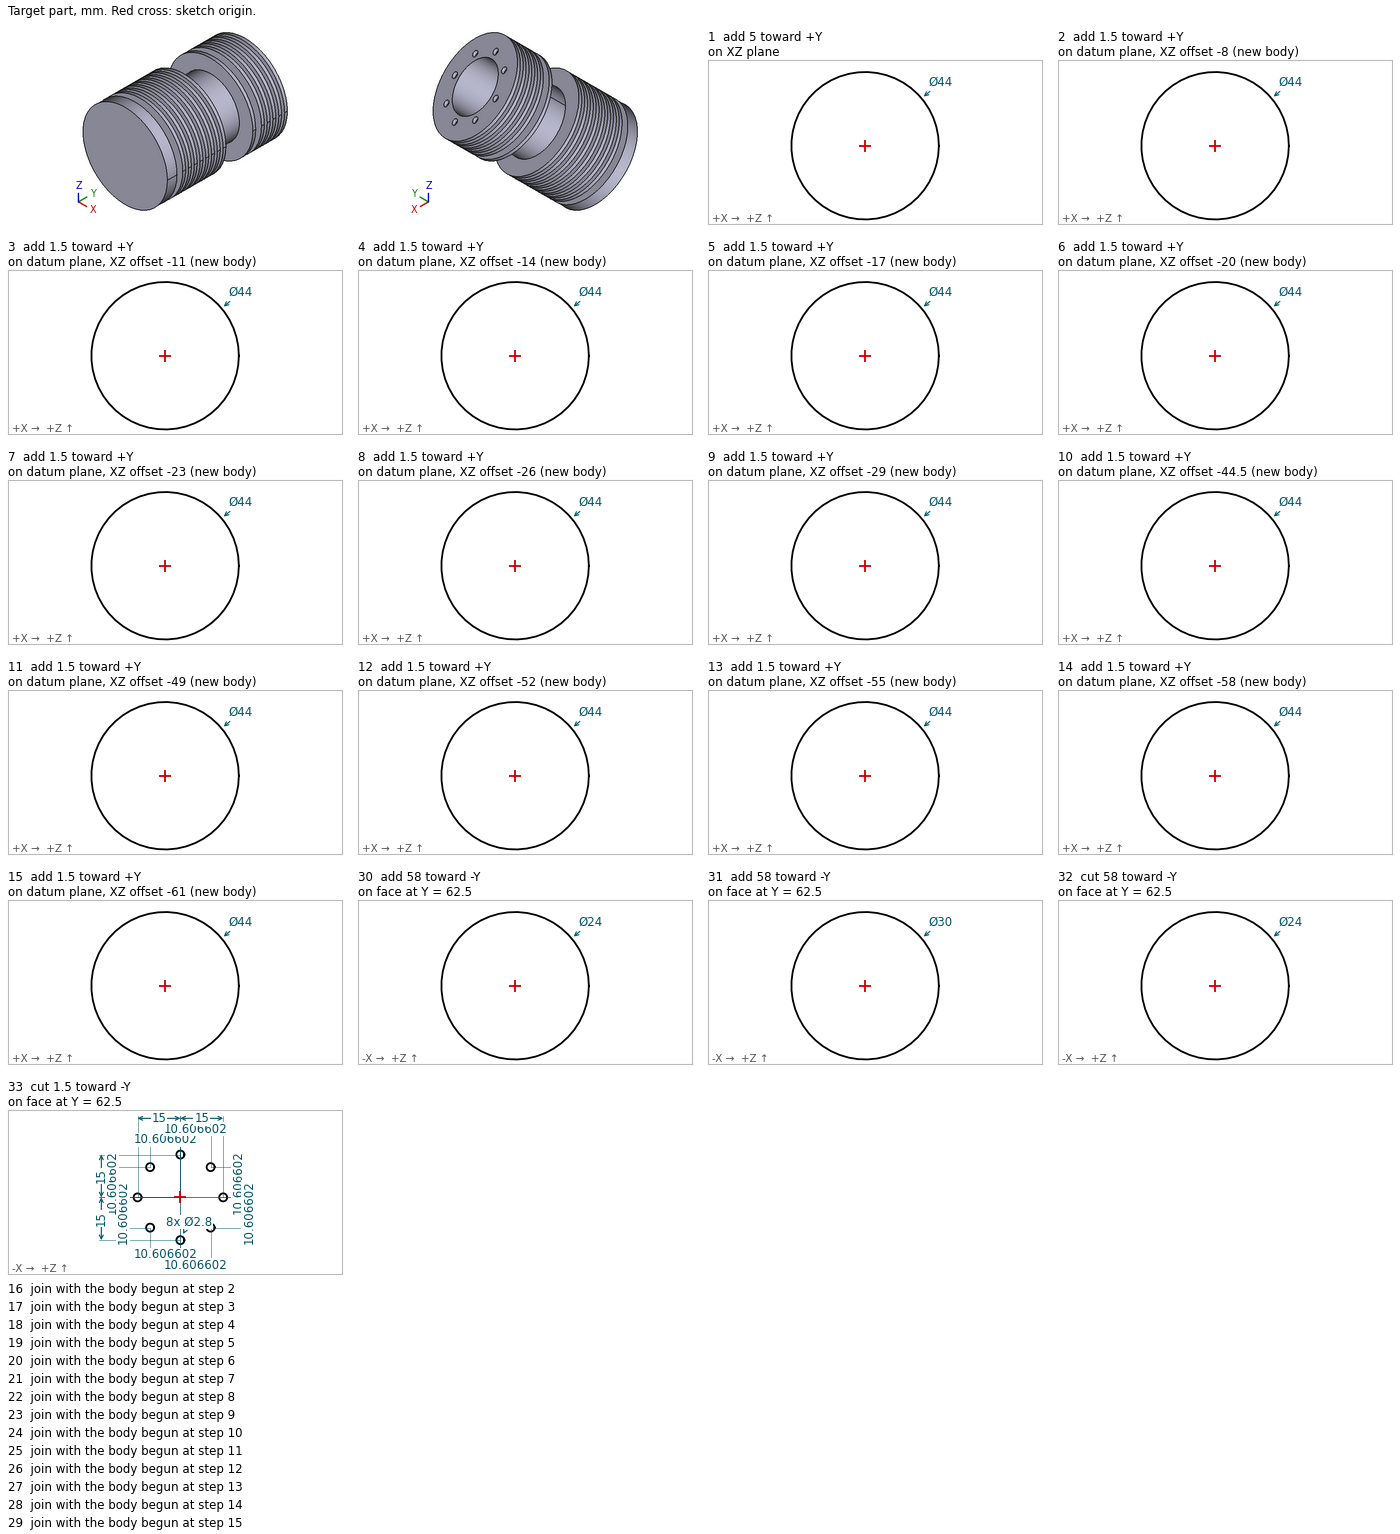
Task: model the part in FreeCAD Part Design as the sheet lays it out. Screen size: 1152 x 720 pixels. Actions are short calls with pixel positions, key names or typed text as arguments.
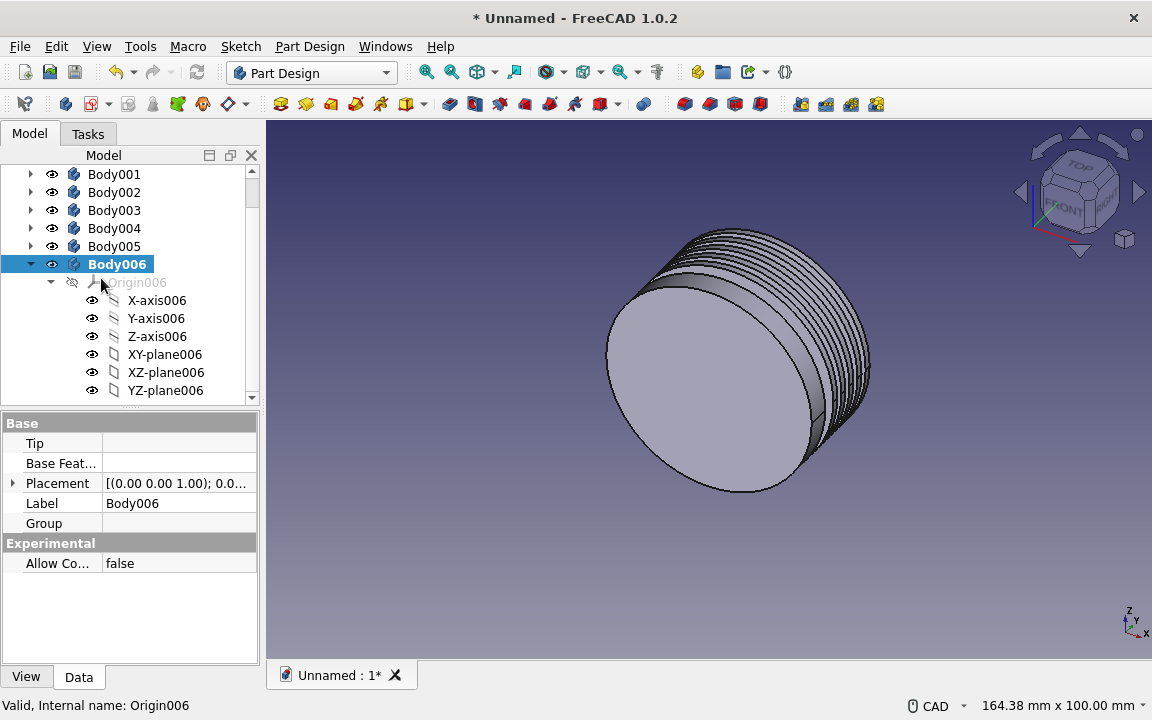
click(137, 372)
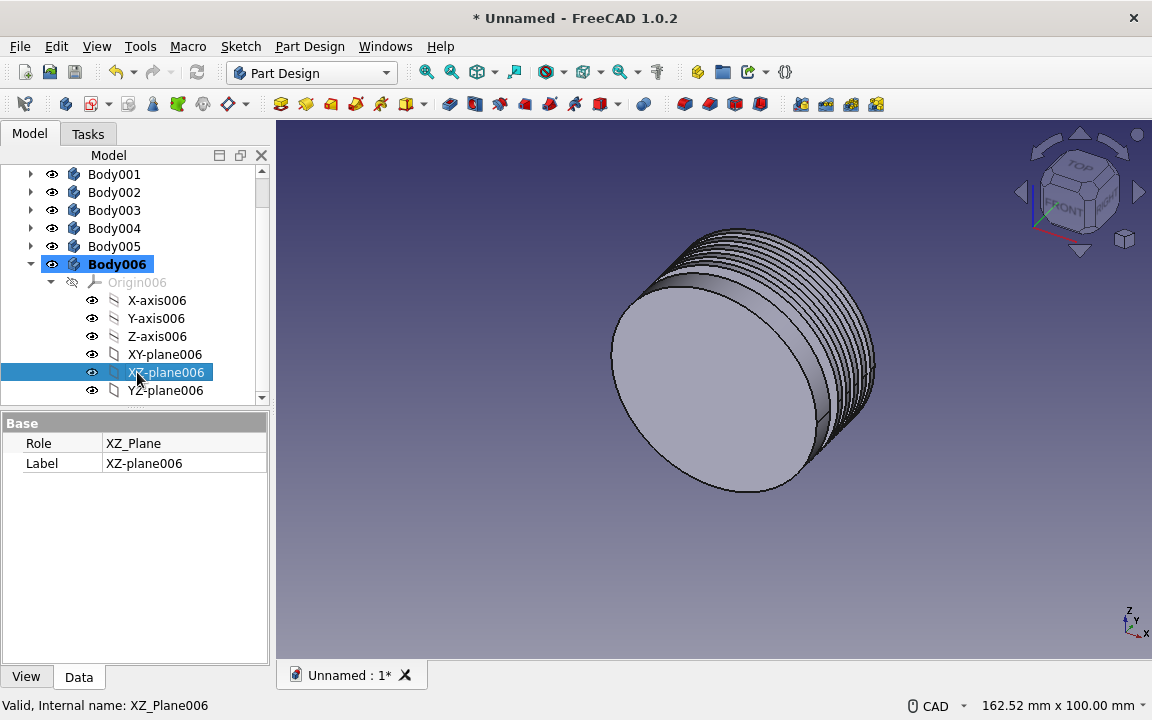
click(228, 104)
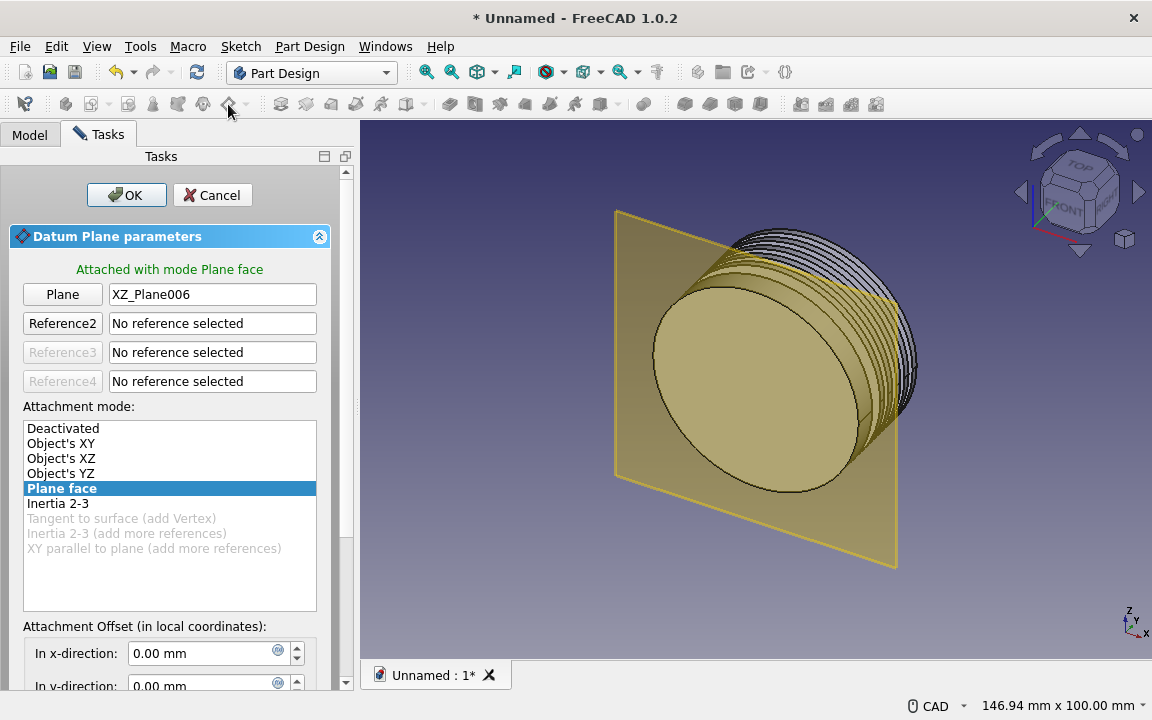
scroll(346, 428, down, 2)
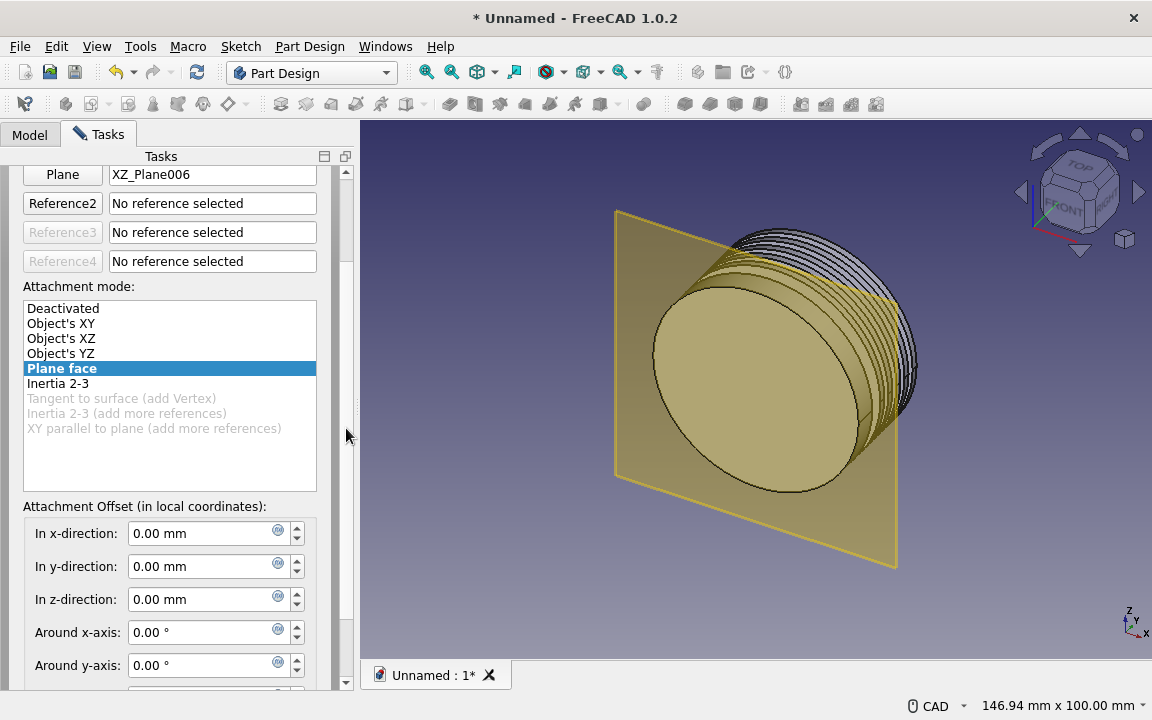
triple_click(210, 600)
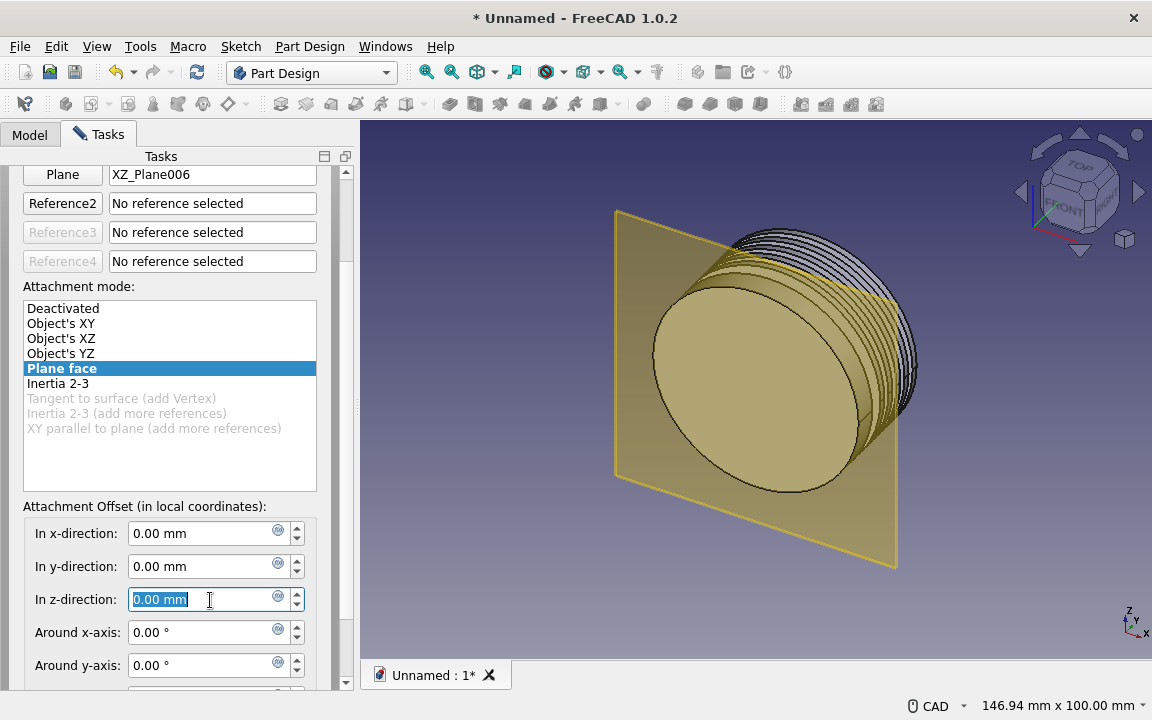
text(-23)
key(Tab)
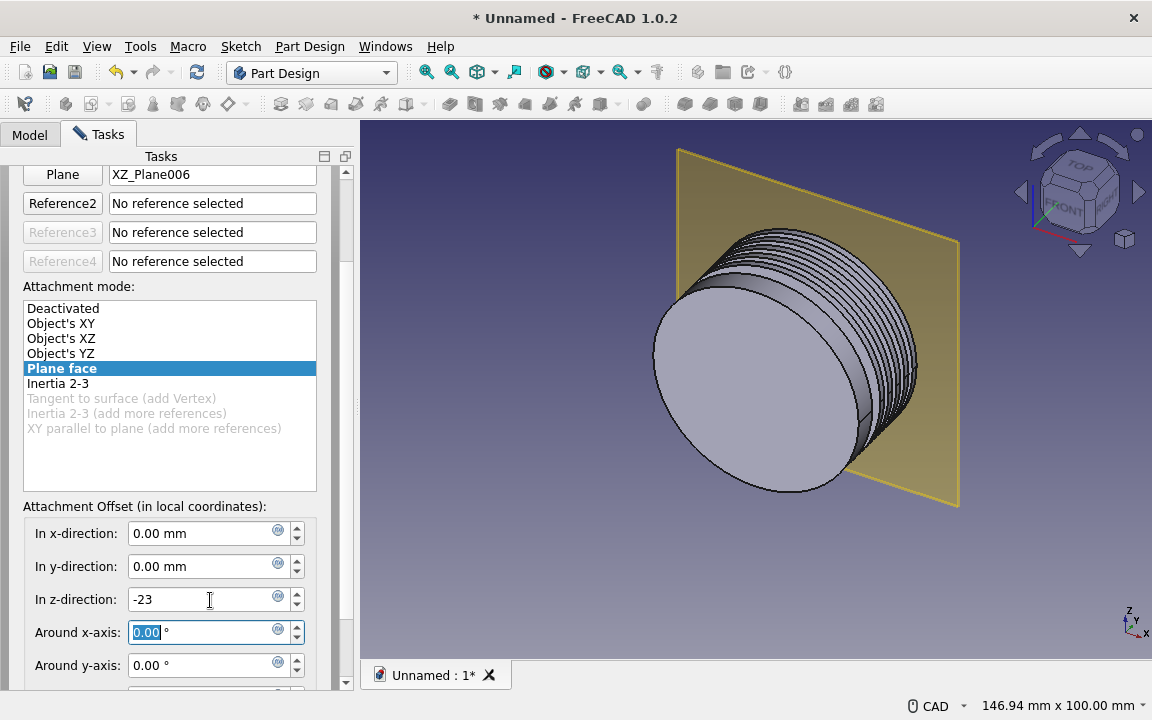
scroll(346, 428, up, 3)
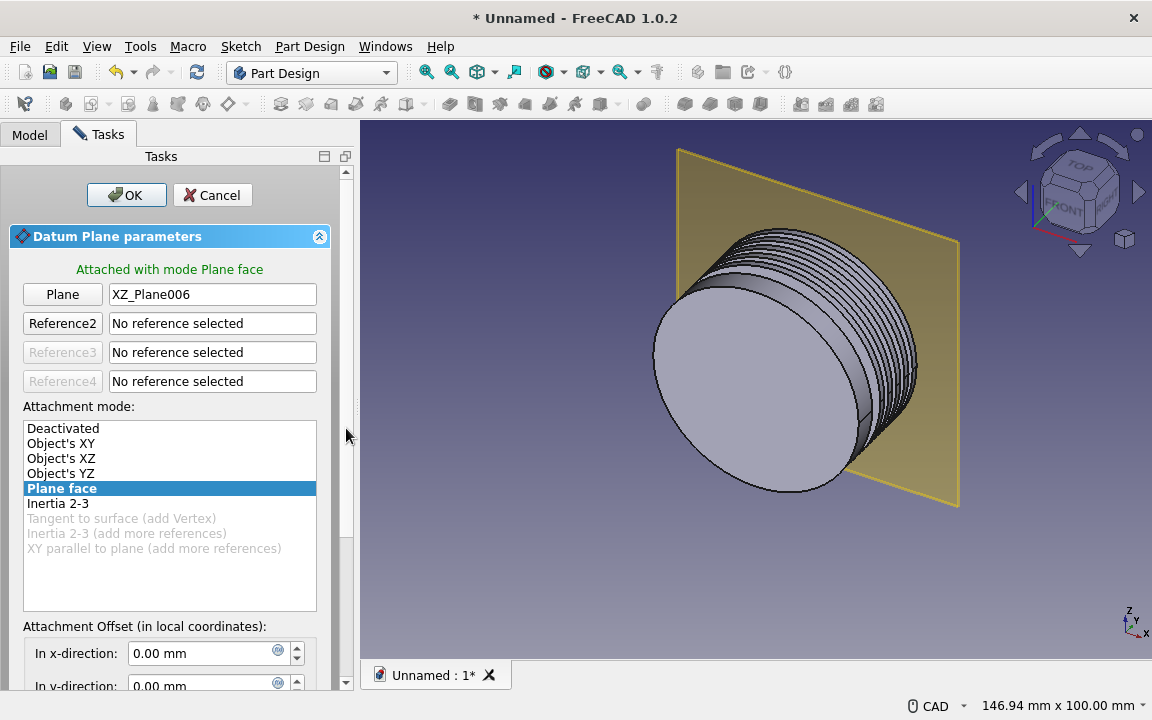
click(127, 195)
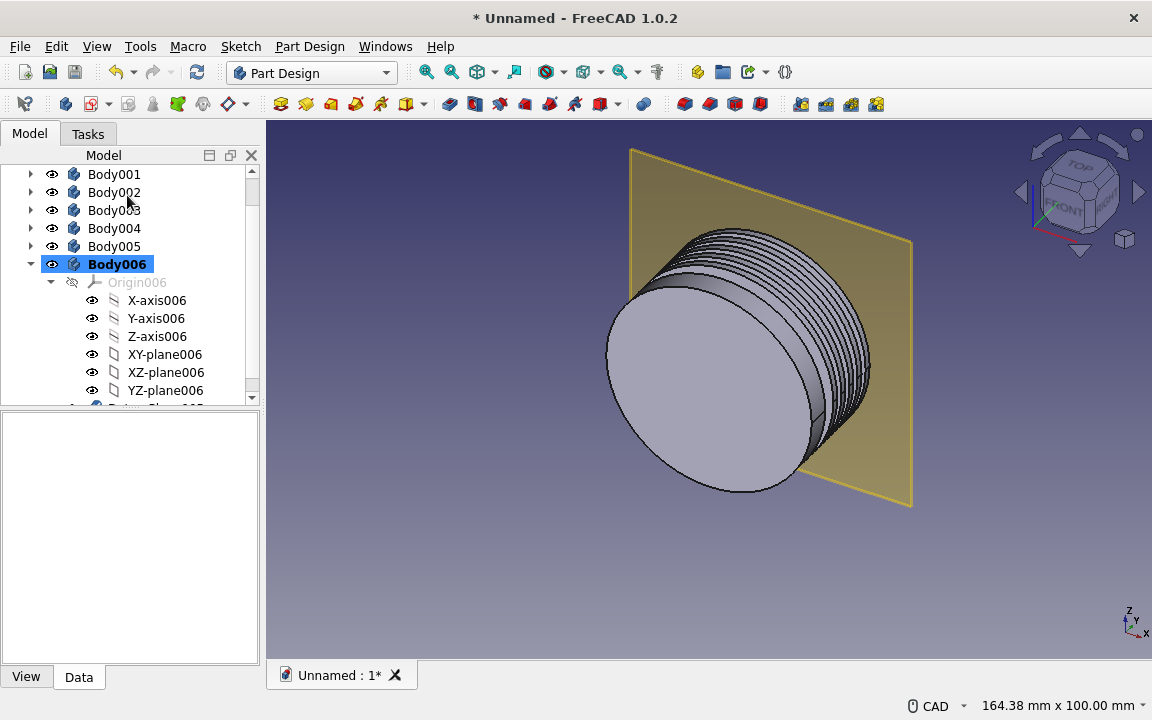
scroll(121, 278, down, 3)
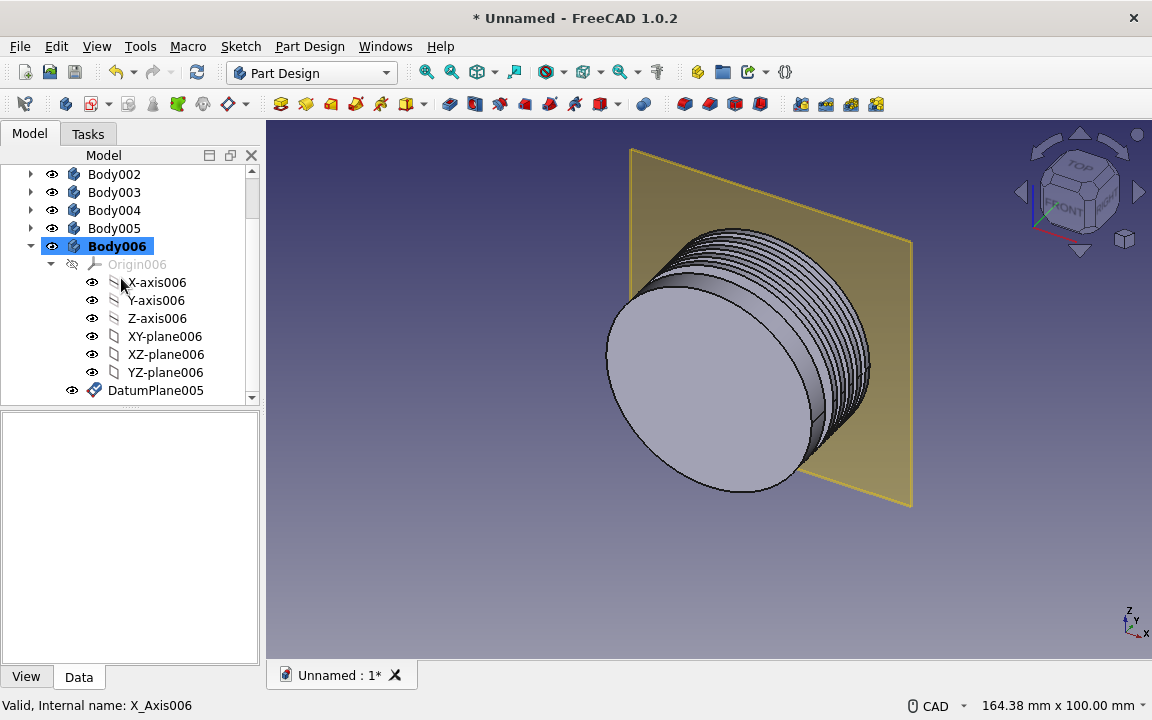
click(117, 390)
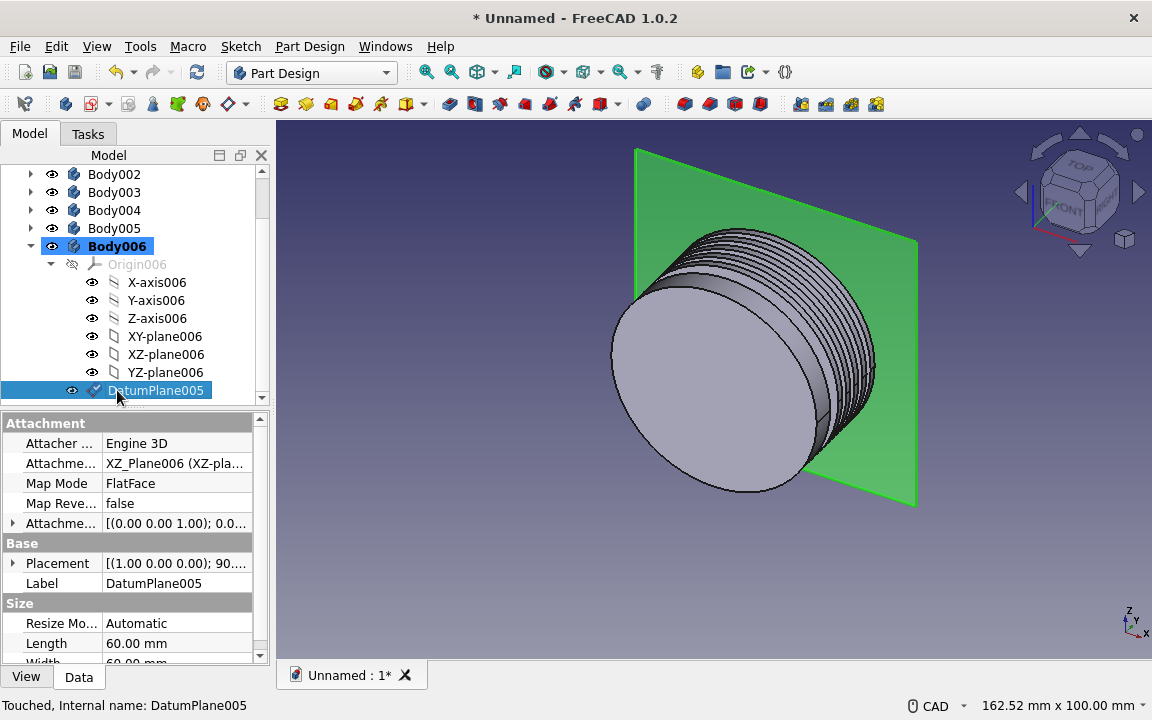
click(90, 104)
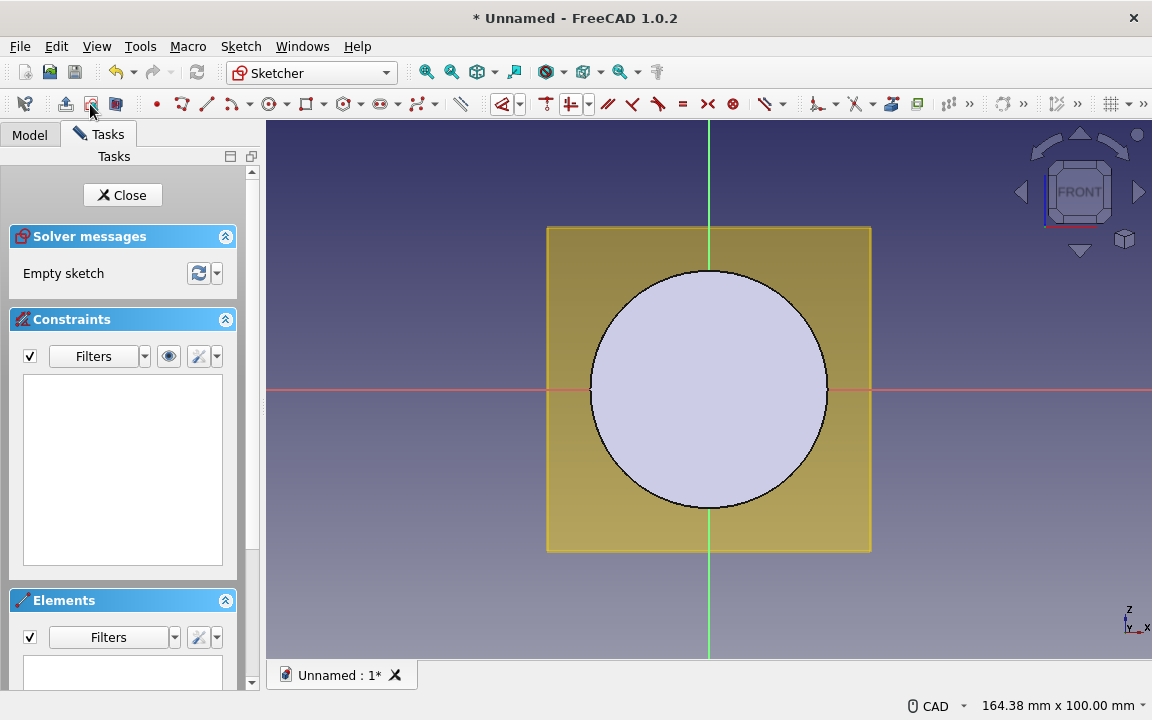
scroll(848, 390, up, 2)